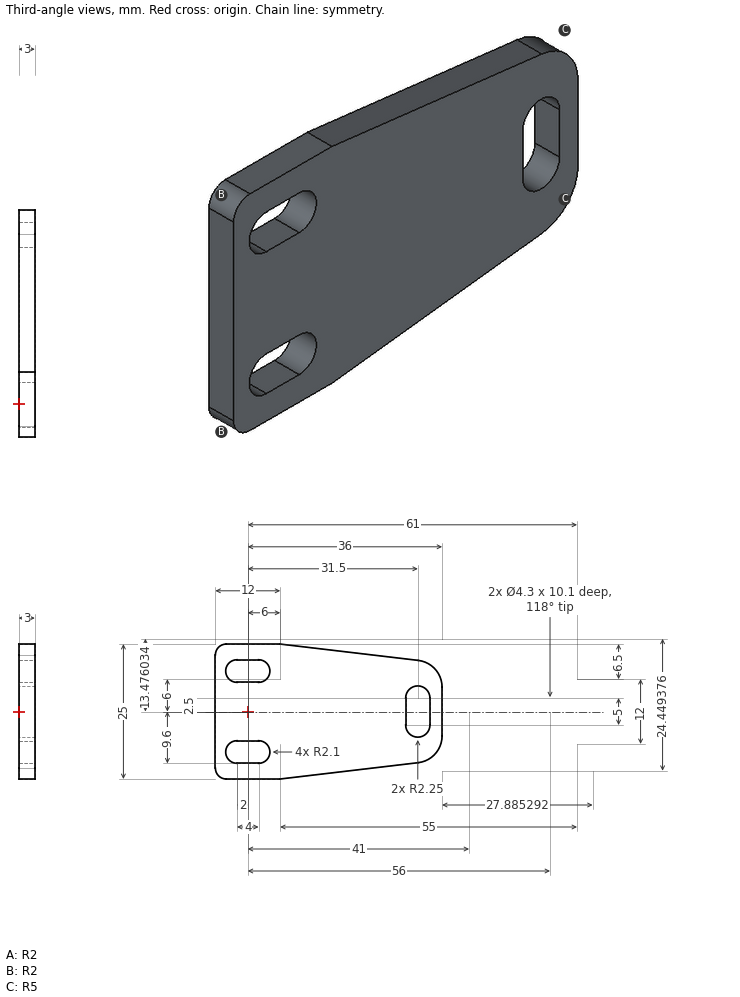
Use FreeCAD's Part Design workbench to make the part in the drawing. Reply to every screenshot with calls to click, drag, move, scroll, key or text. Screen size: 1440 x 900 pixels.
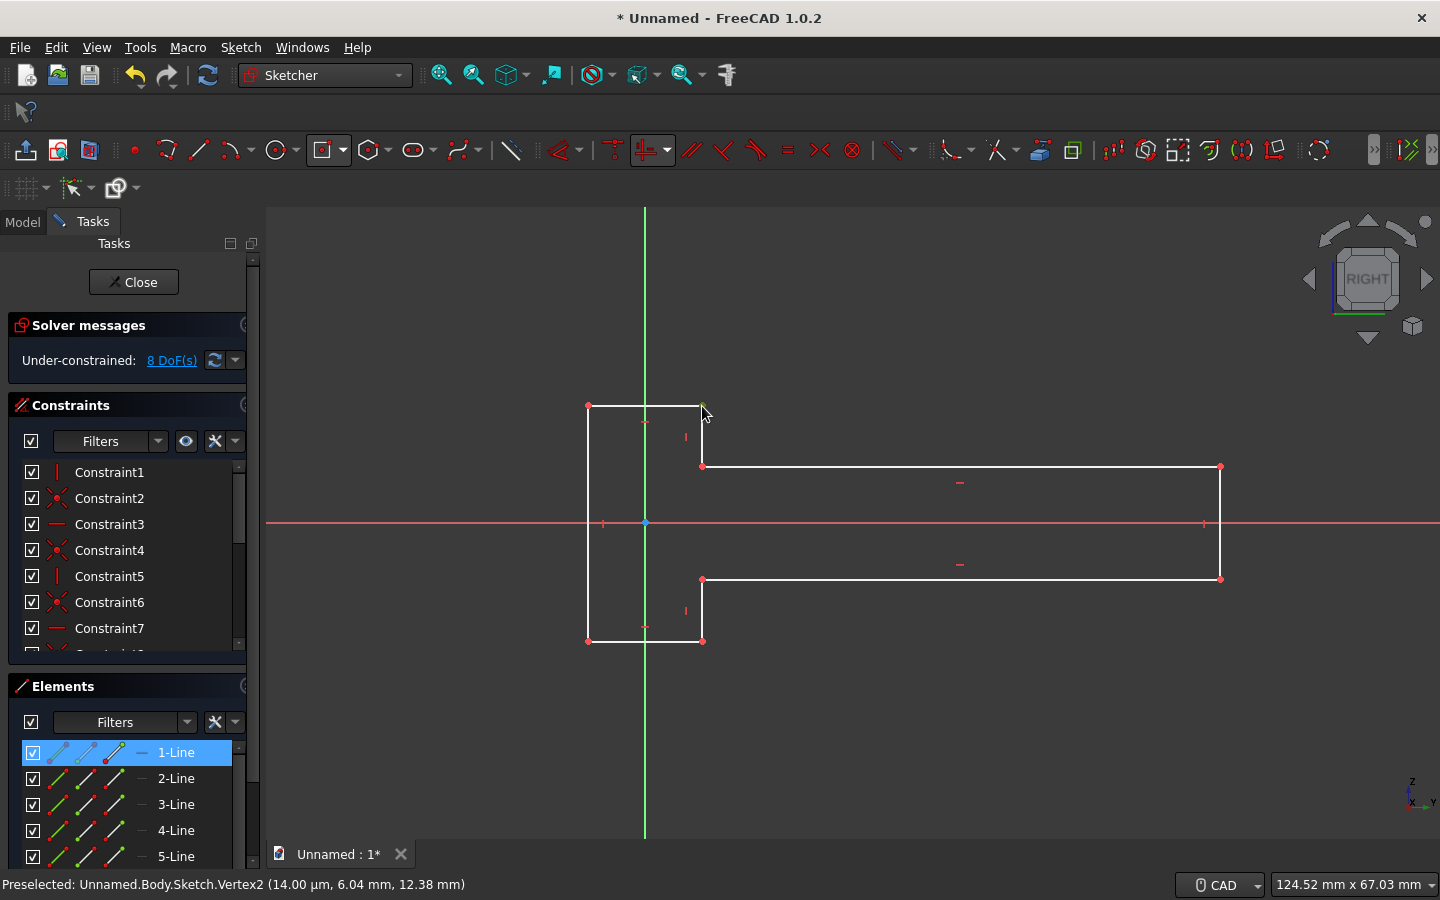
click(702, 642)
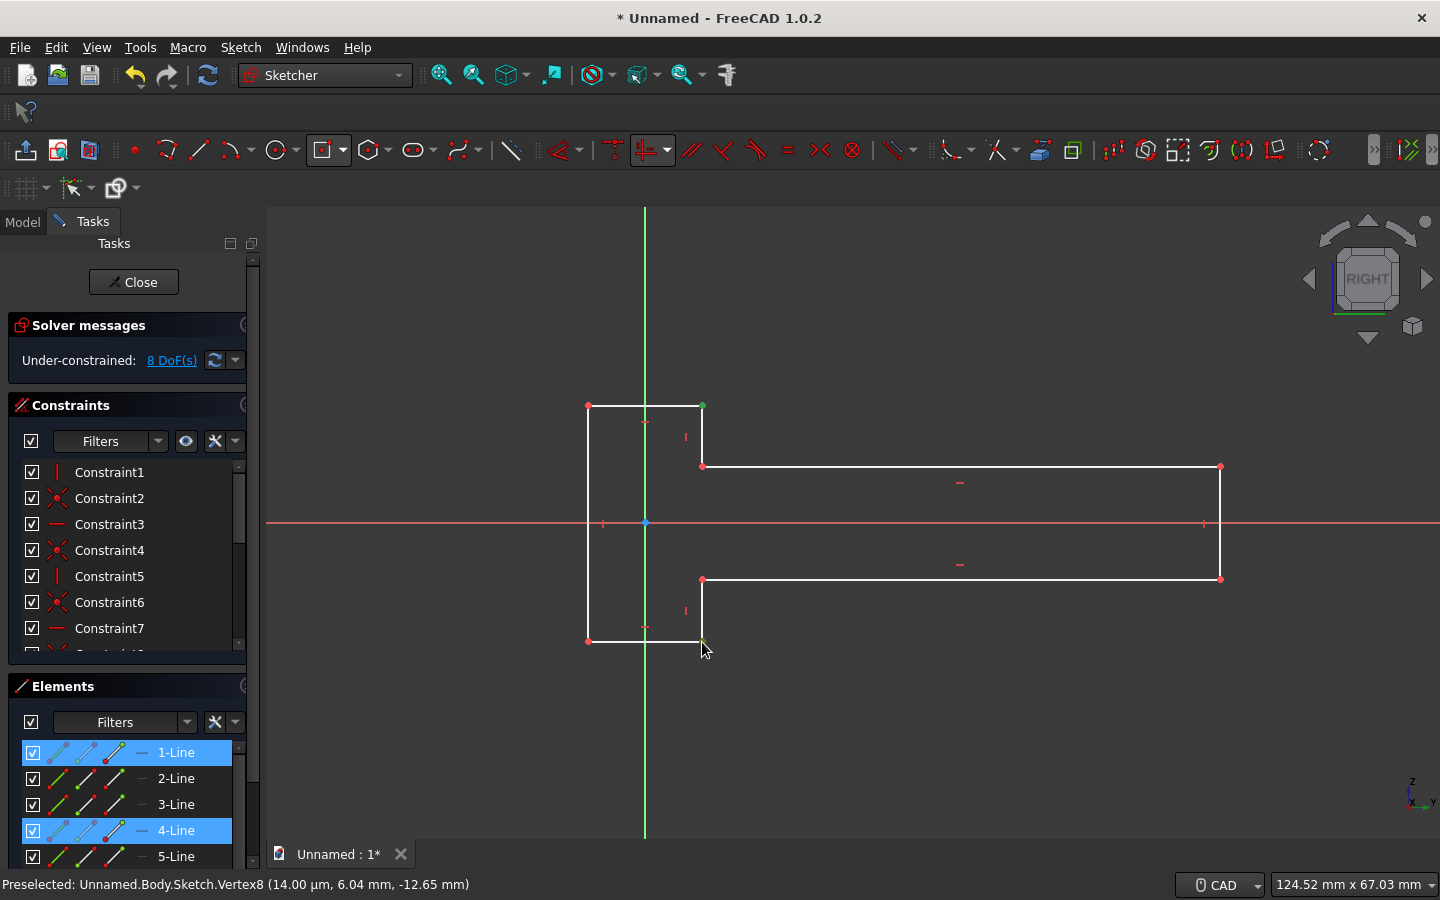
click(364, 523)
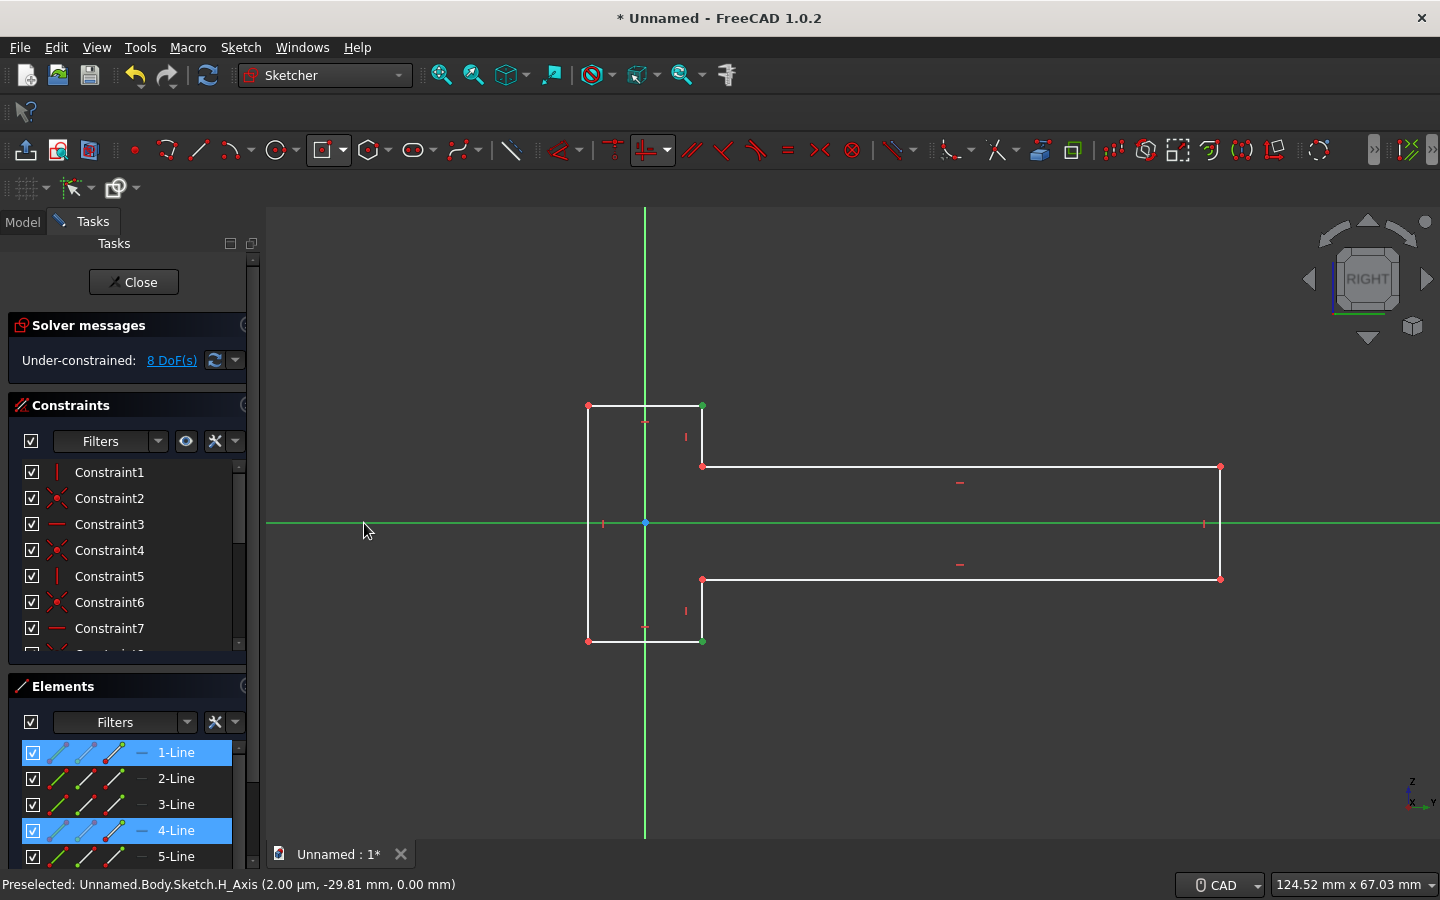
key(s)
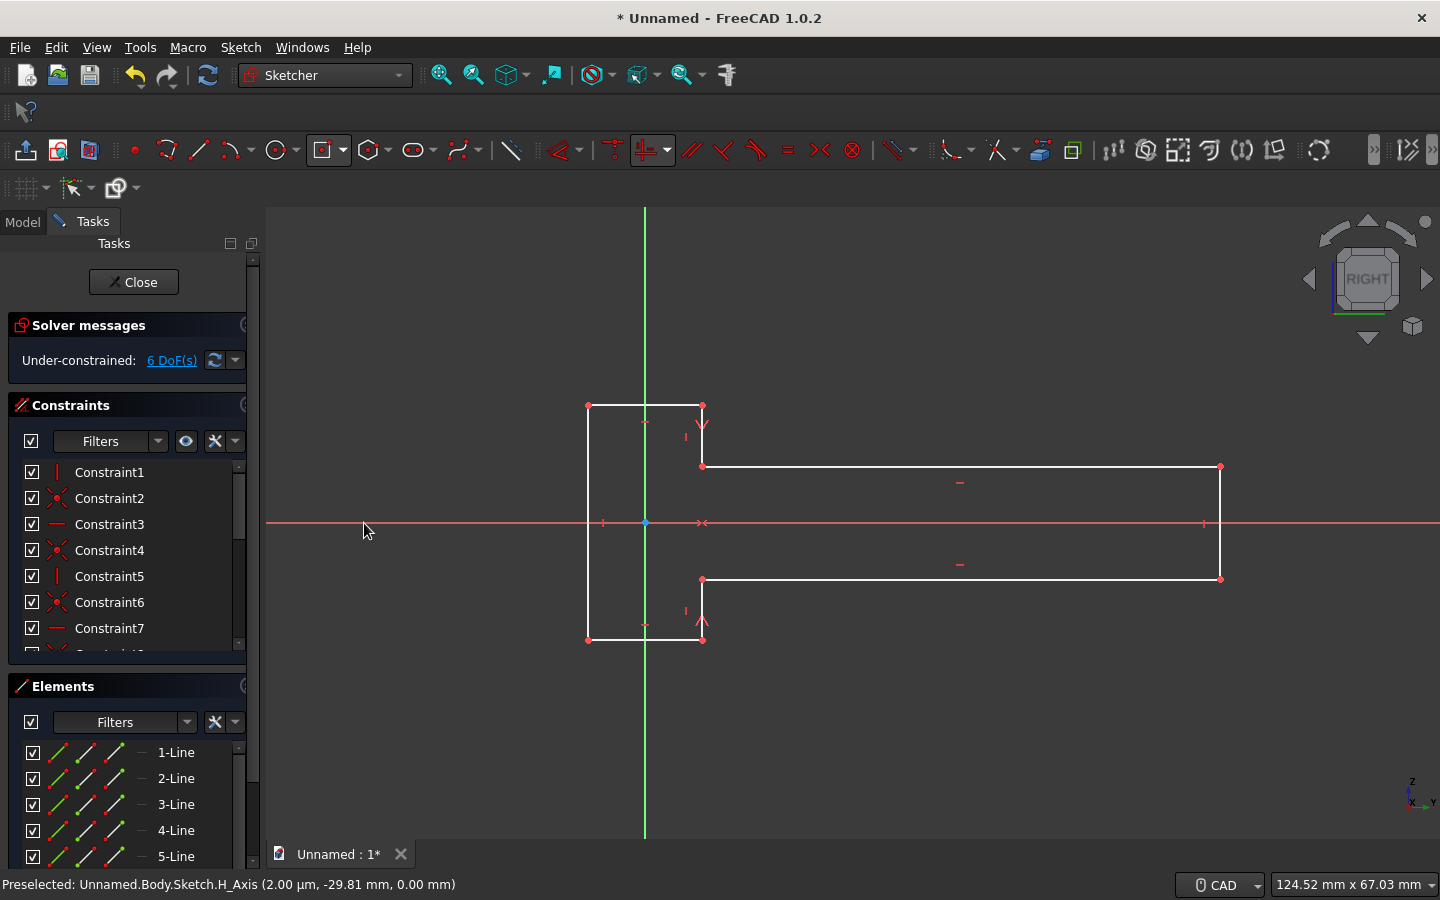
key(d)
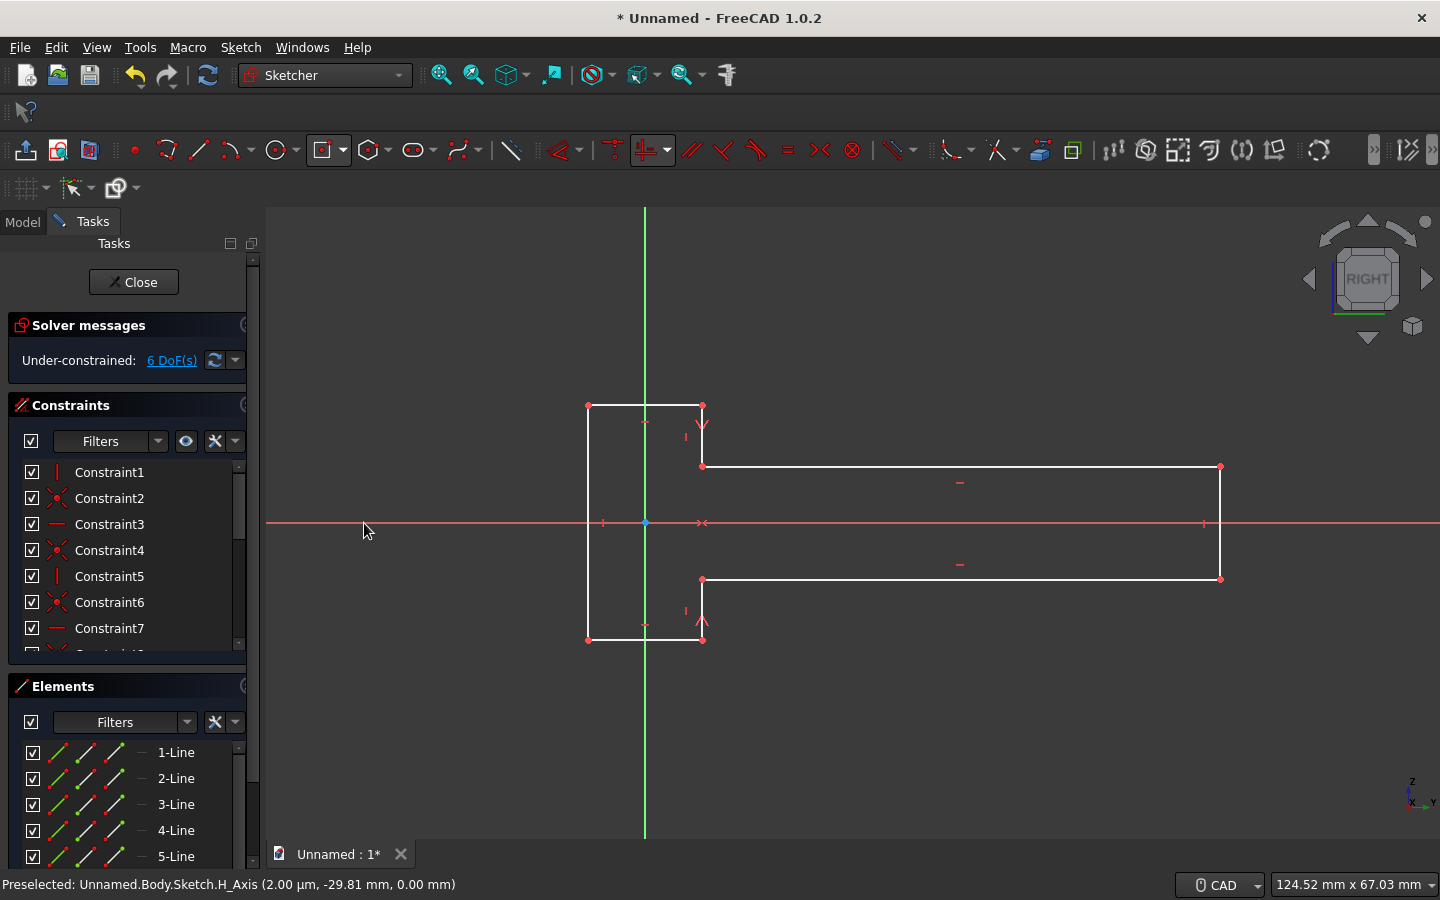
click(668, 405)
click(619, 371)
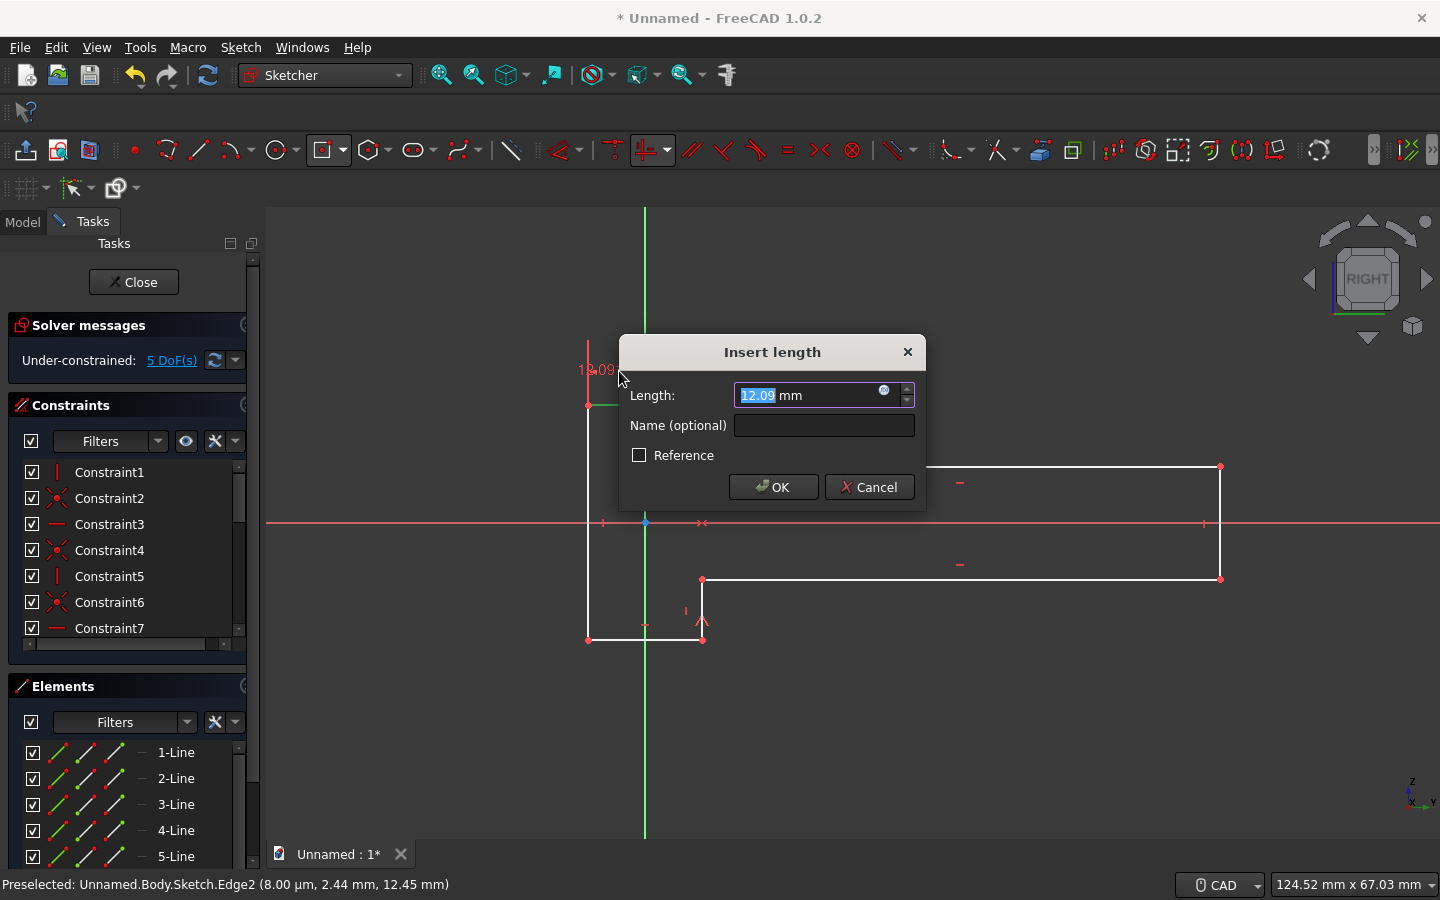
text(12)
key(Return)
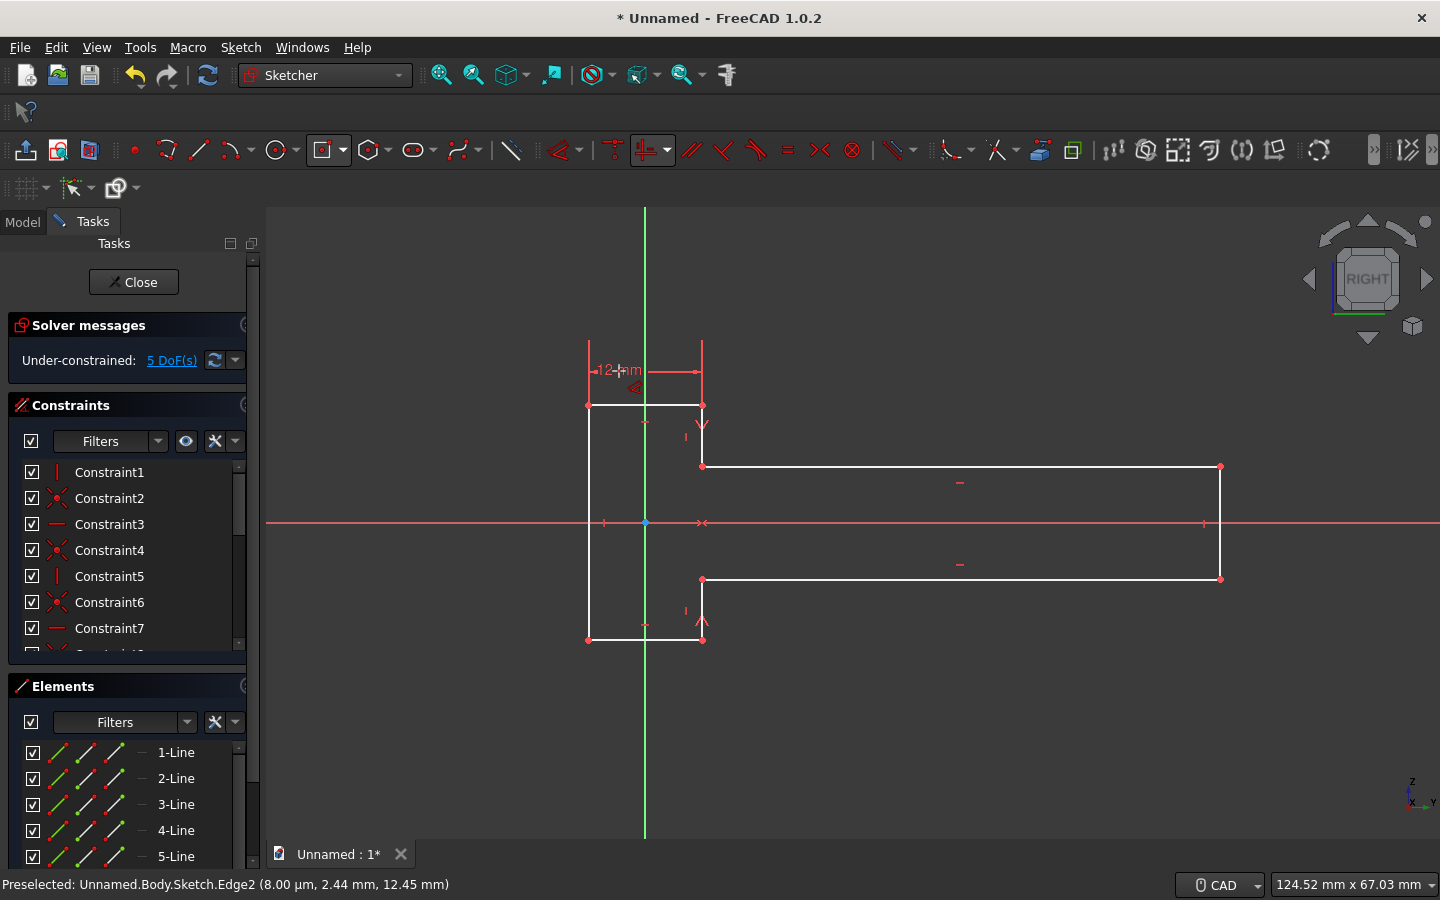
click(589, 476)
click(555, 469)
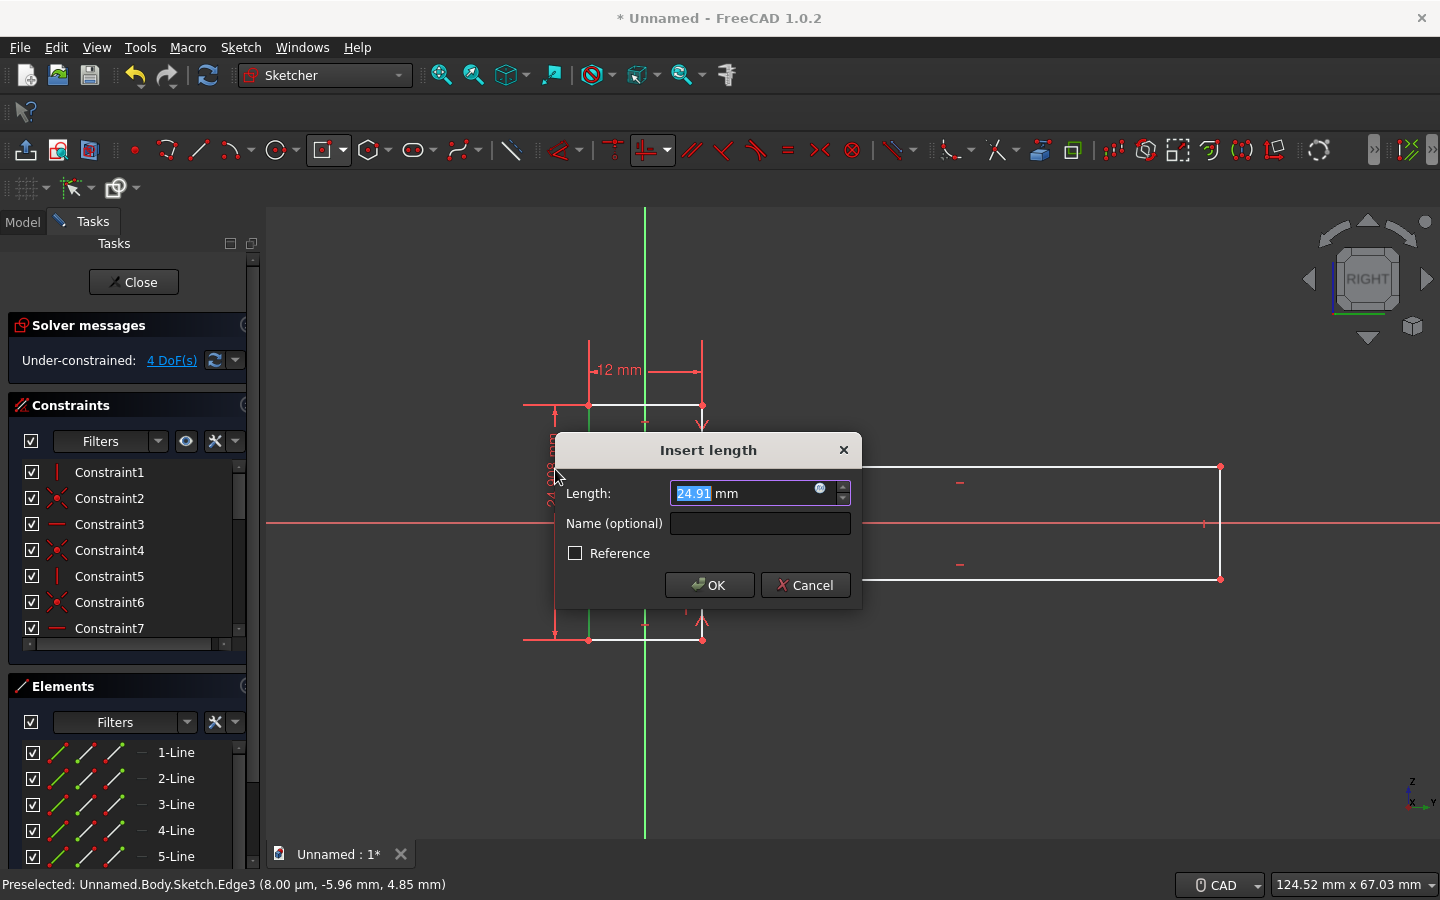
text(25)
key(Return)